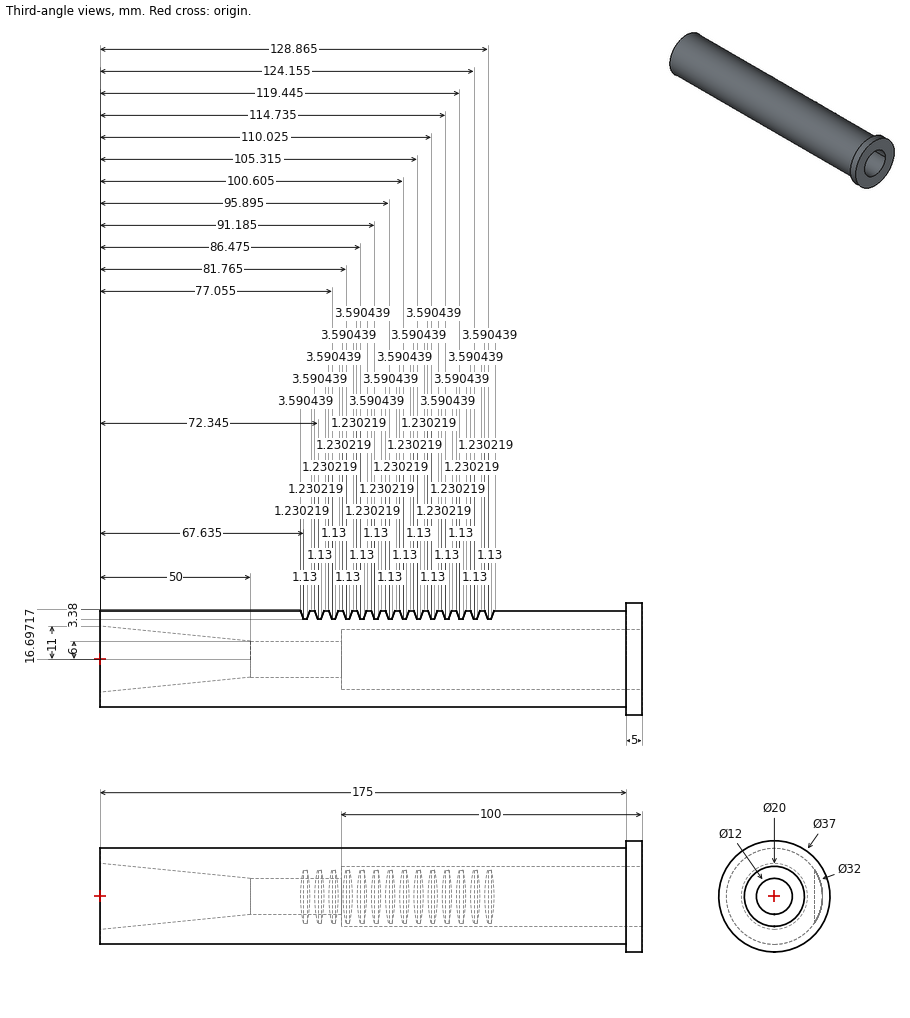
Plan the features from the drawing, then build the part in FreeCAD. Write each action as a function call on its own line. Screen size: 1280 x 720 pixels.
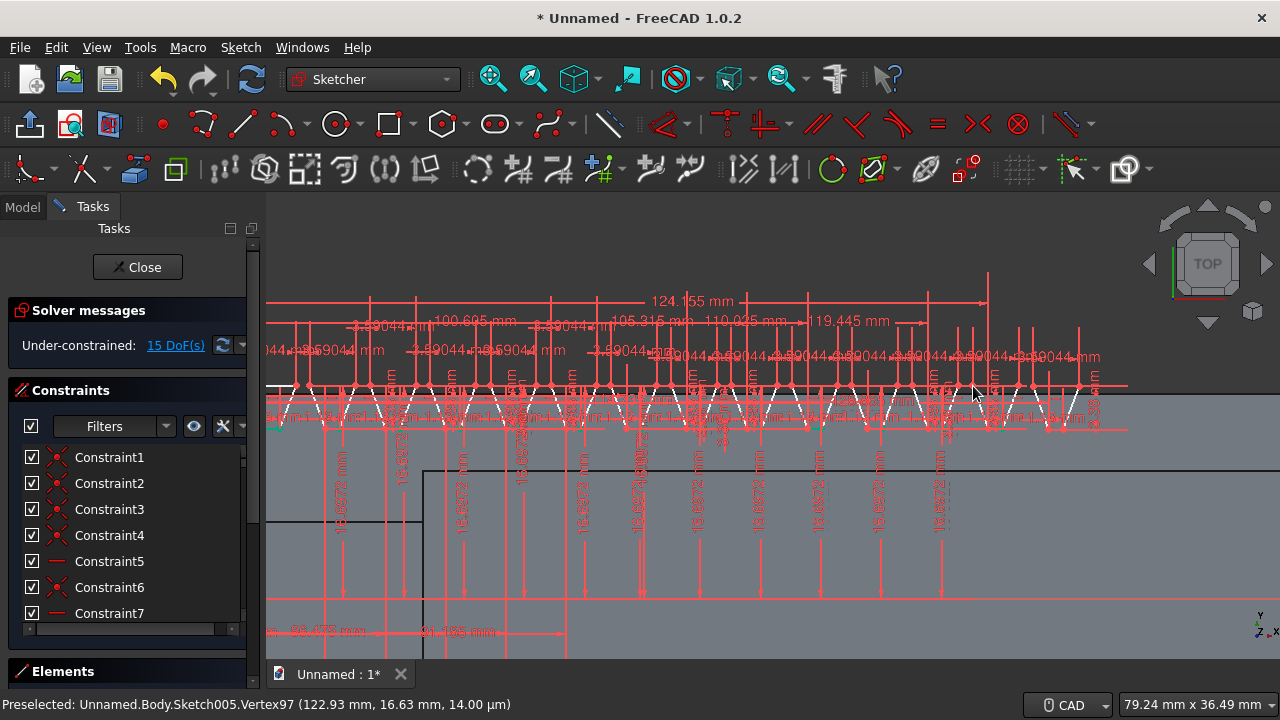
click(1033, 386)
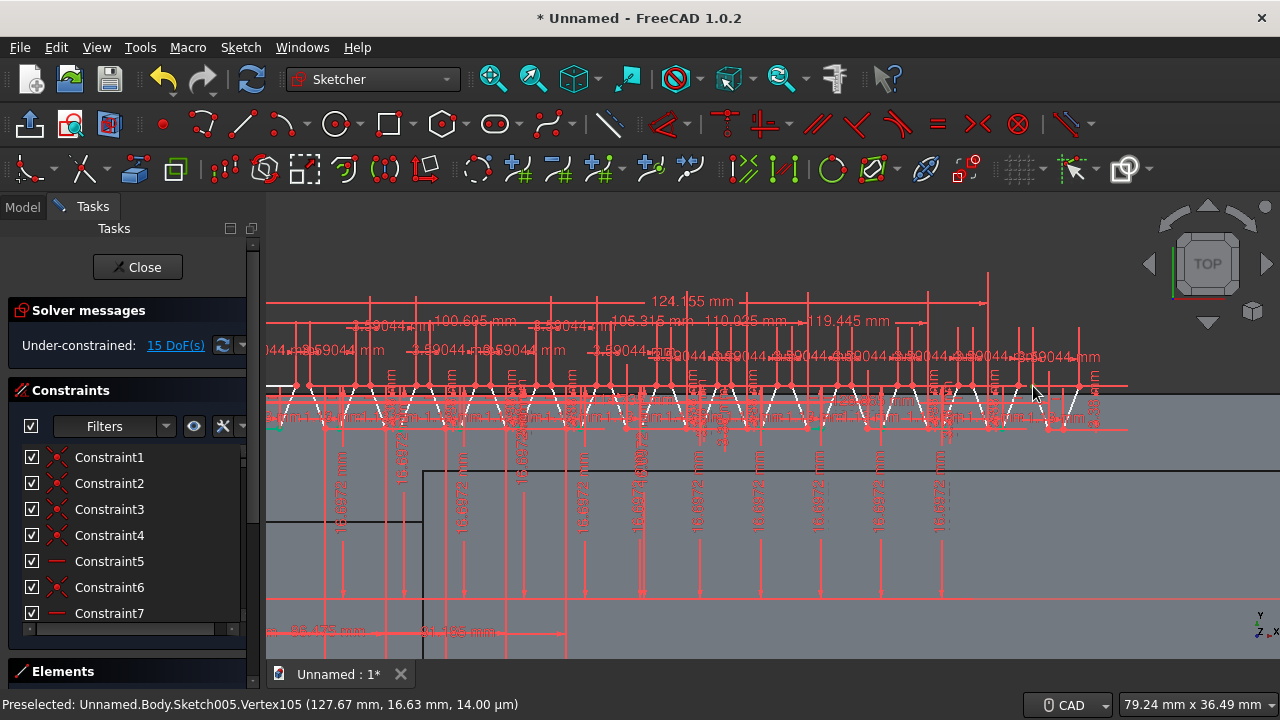
click(690, 124)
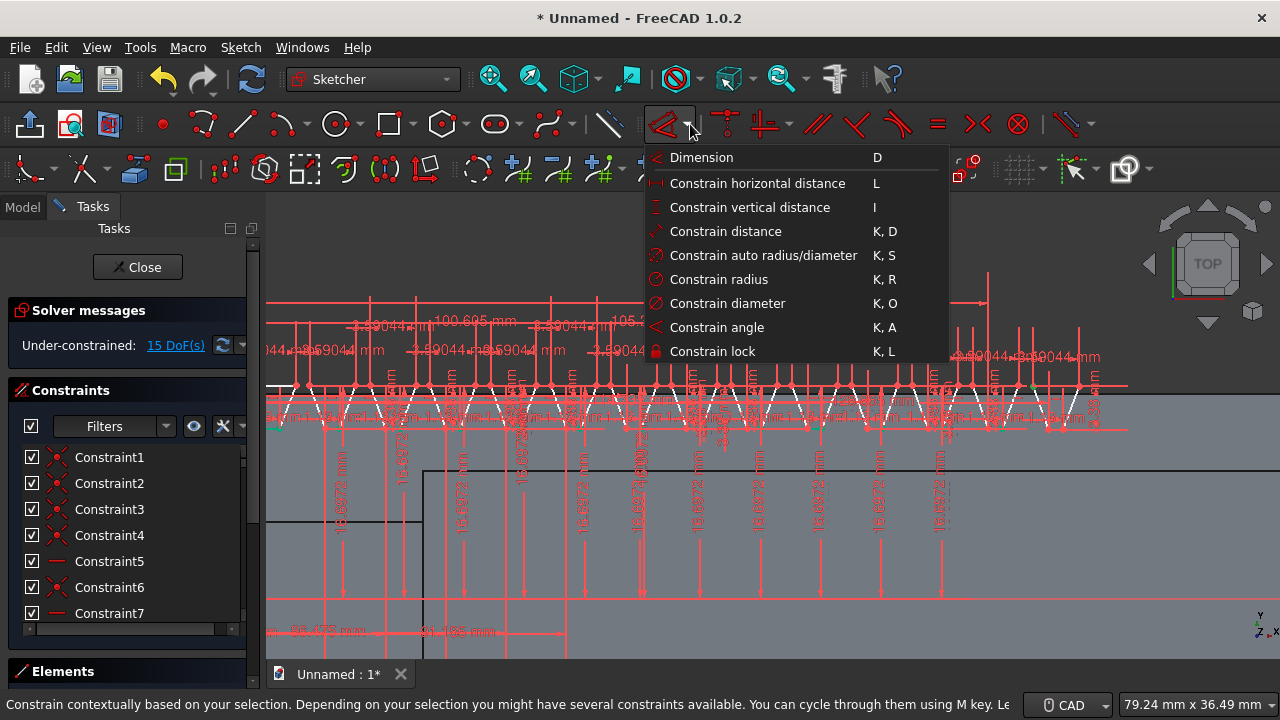
click(797, 207)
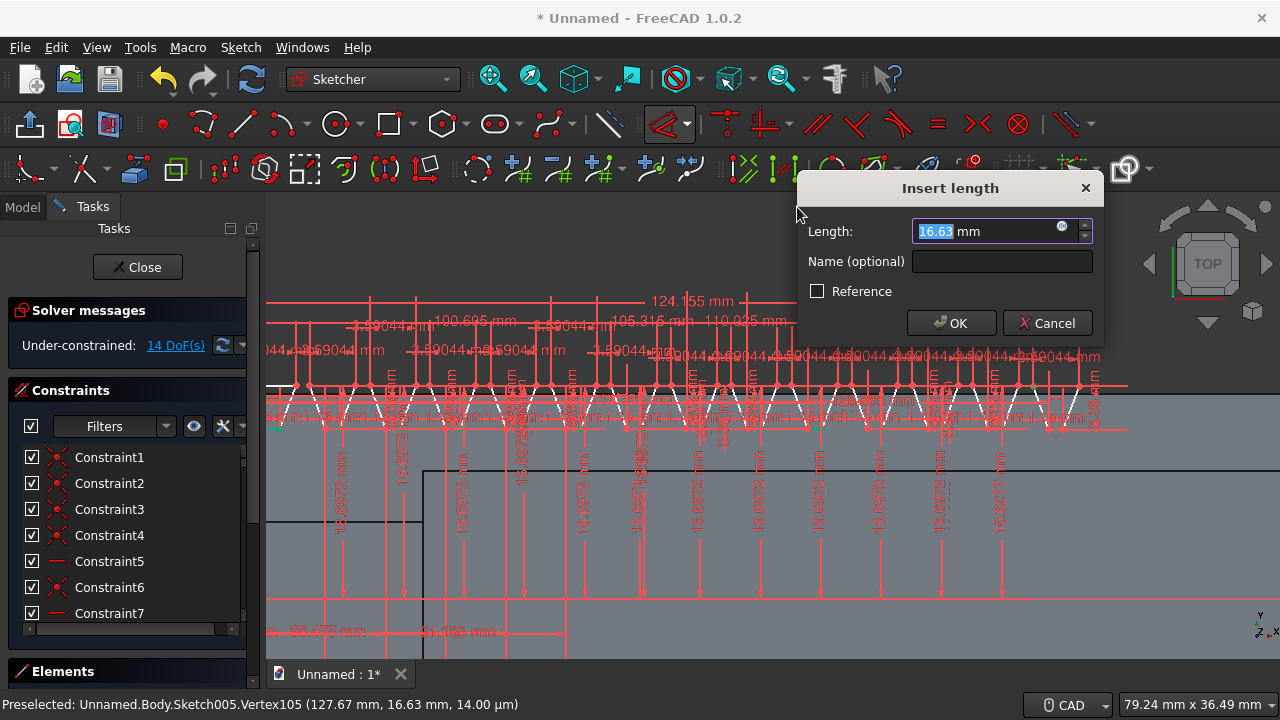
text(16.69717)
key(Return)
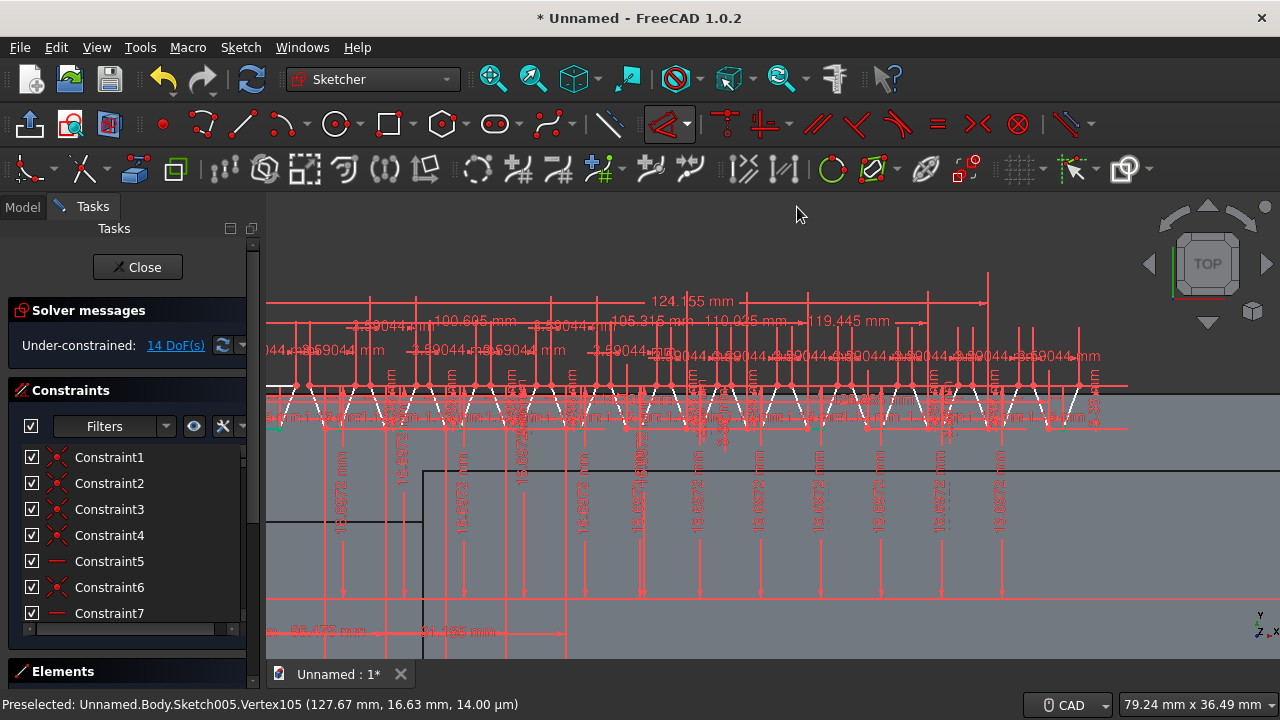
scroll(975, 387, down, 5)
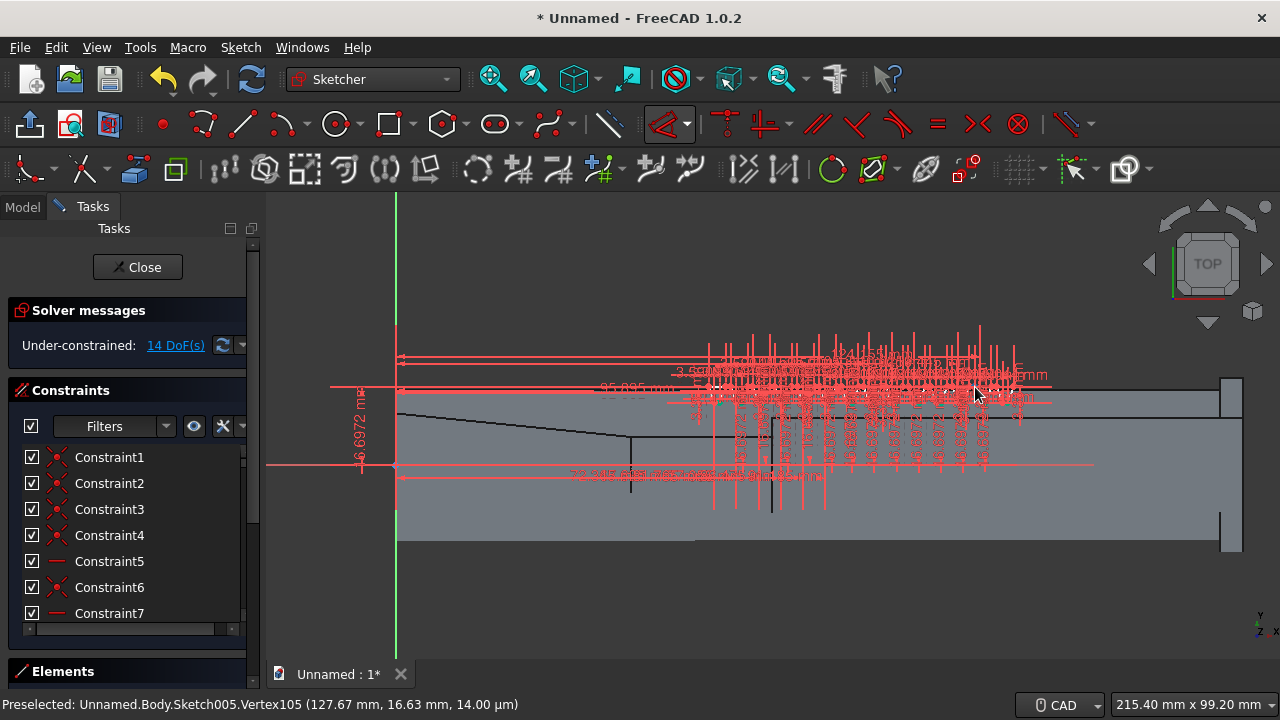
scroll(710, 391, up, 10)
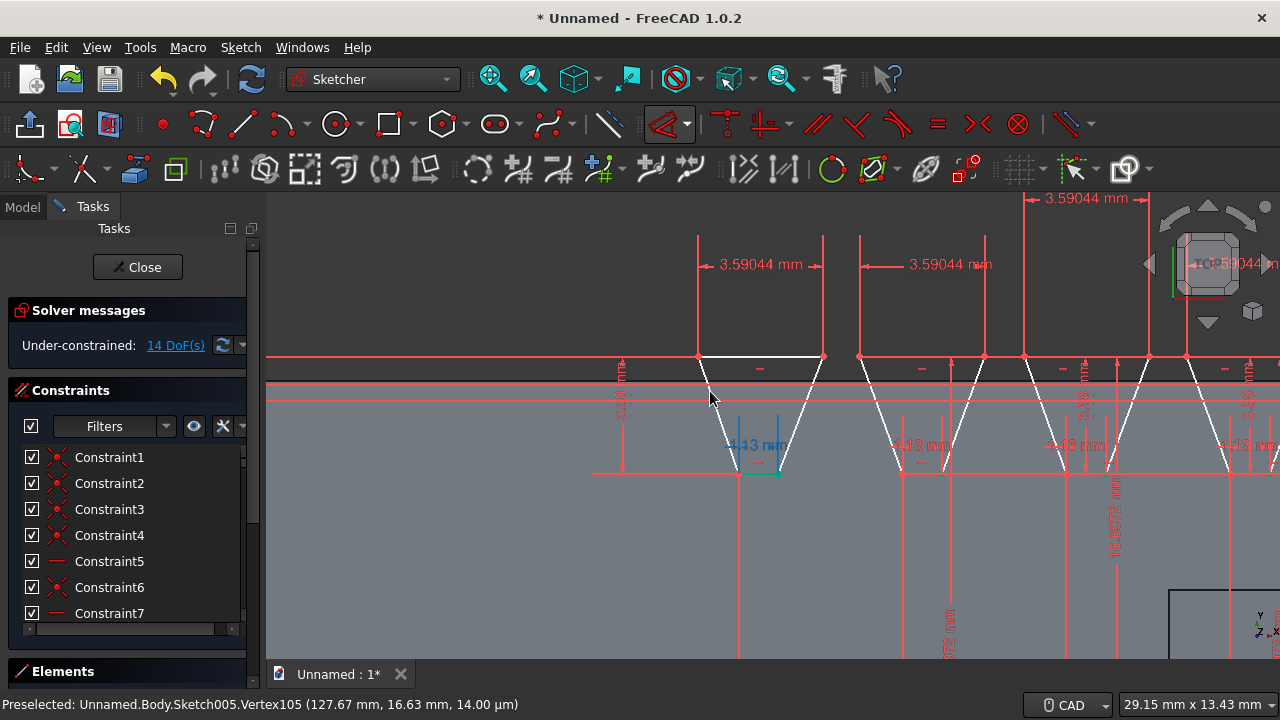
click(710, 392)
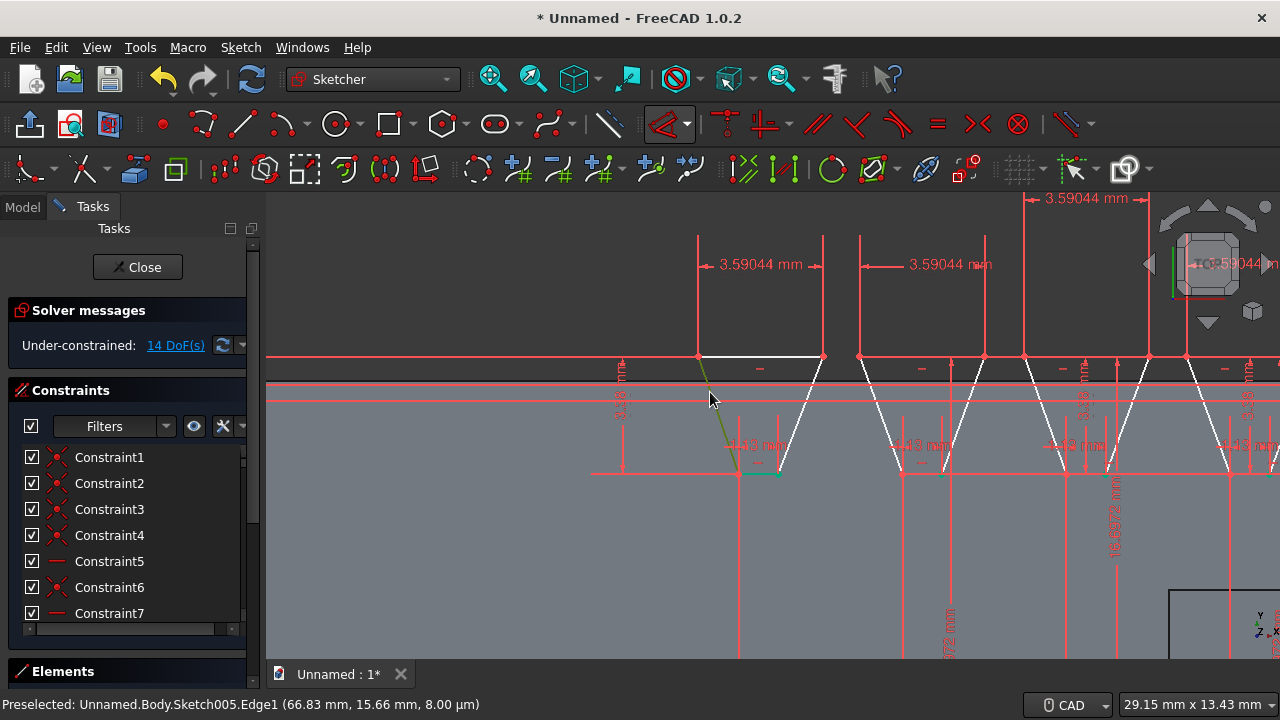
key(l)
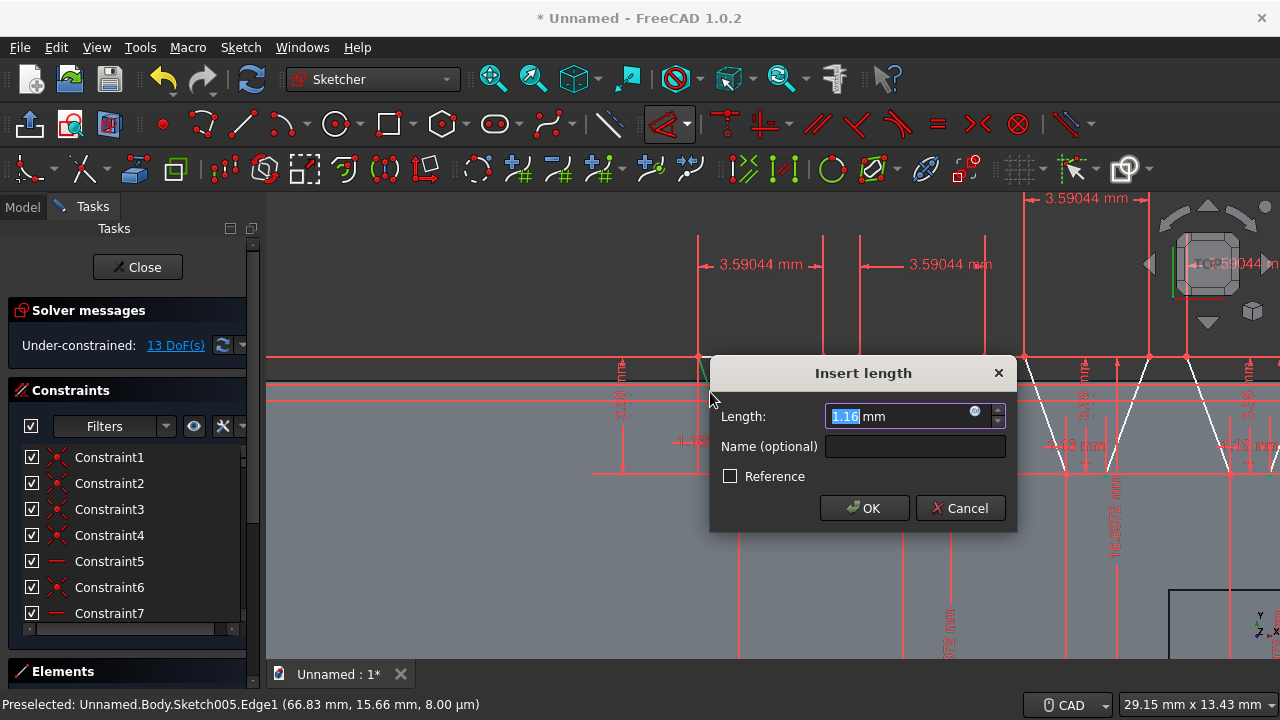
text(1.230219)
key(Return)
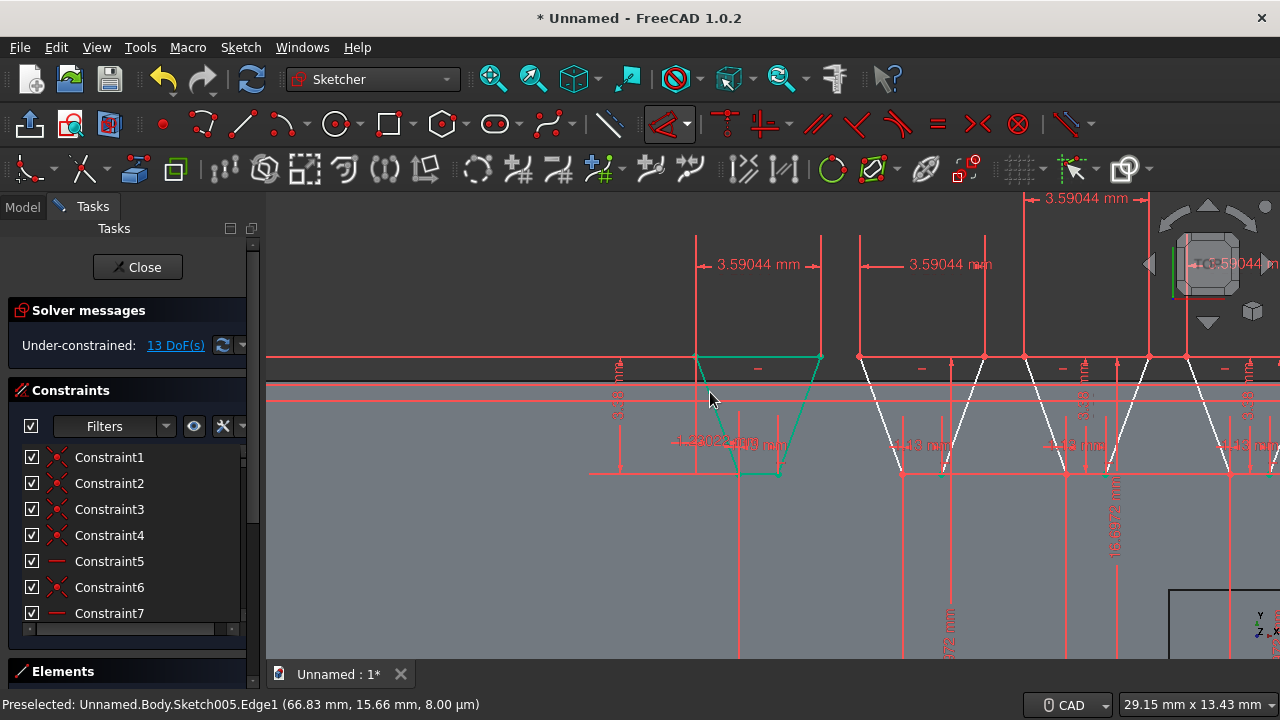
click(873, 392)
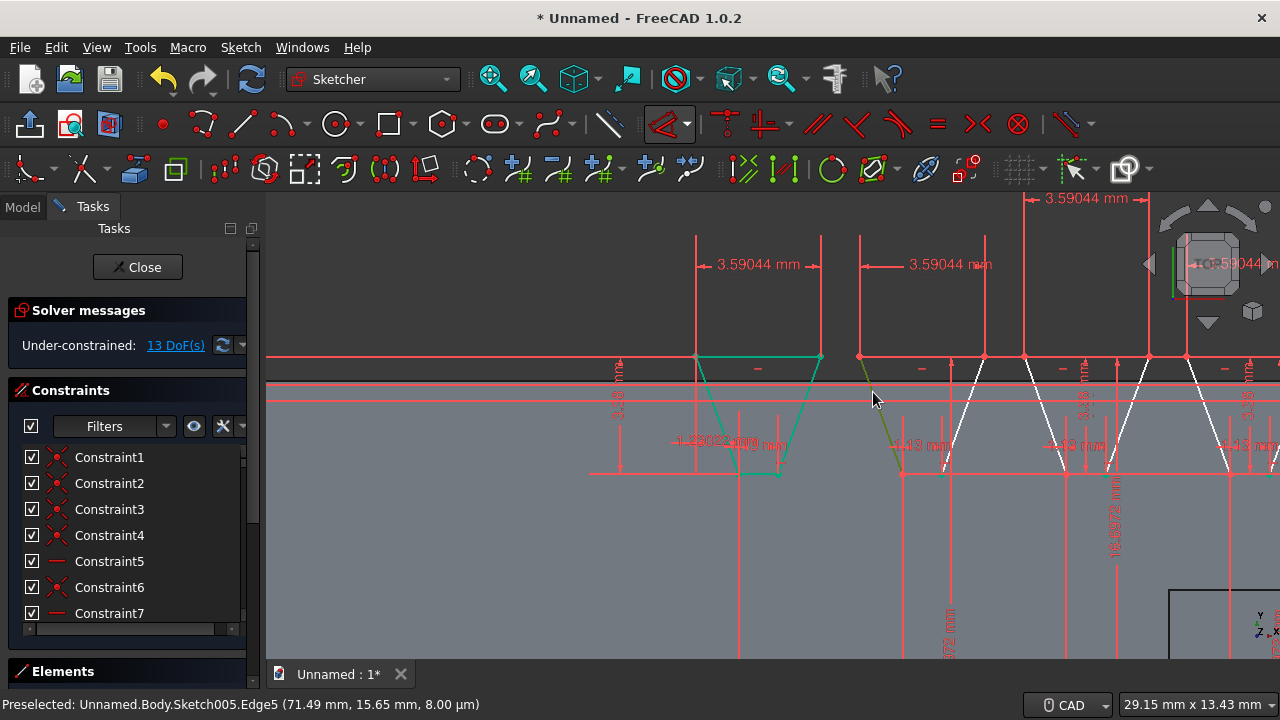
key(l)